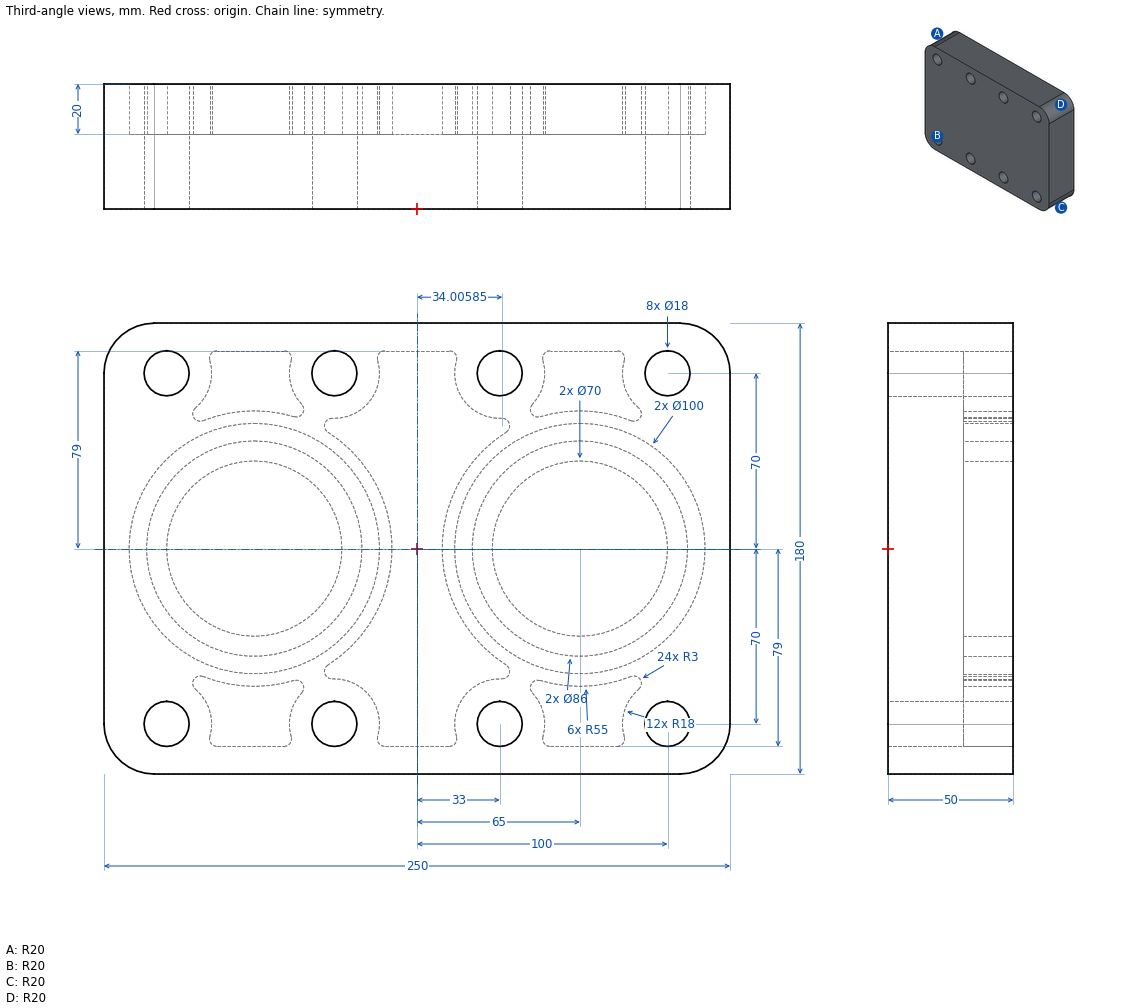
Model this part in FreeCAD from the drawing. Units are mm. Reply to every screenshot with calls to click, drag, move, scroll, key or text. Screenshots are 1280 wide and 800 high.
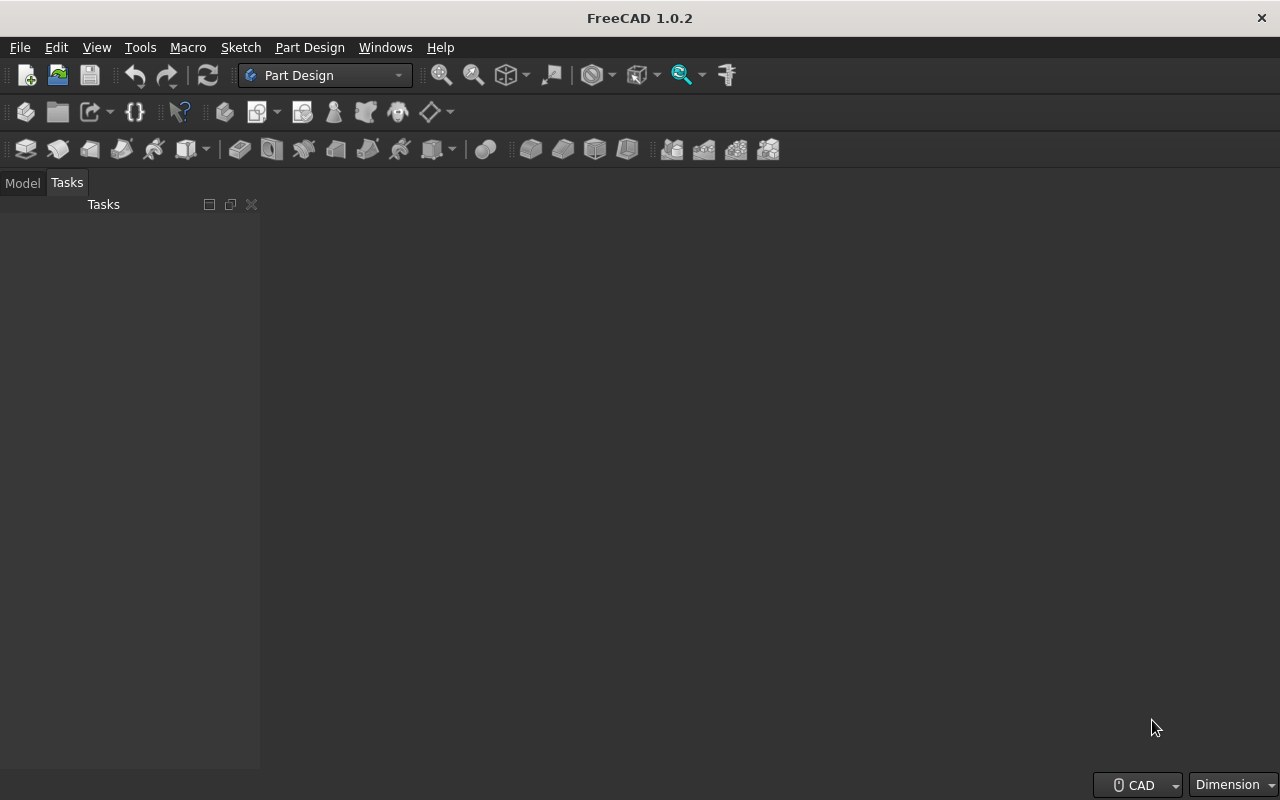
click(26, 76)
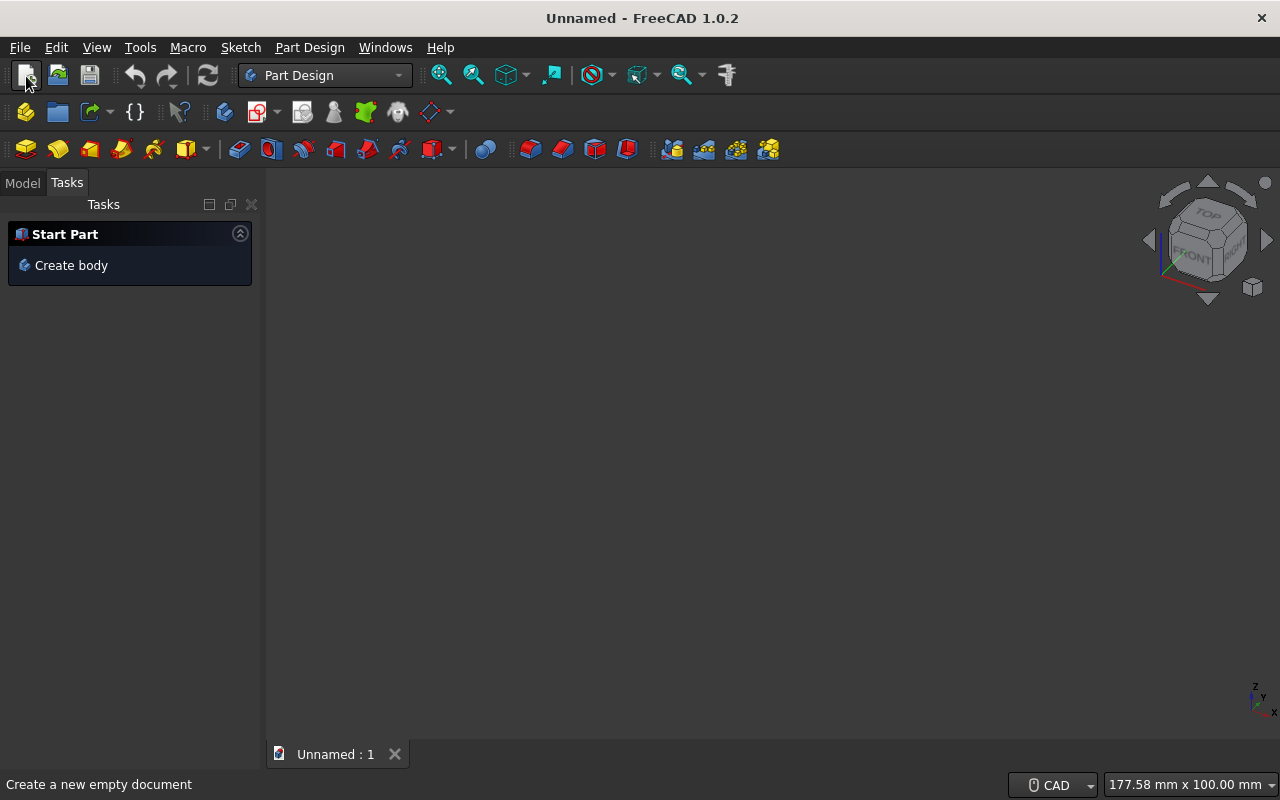
click(258, 112)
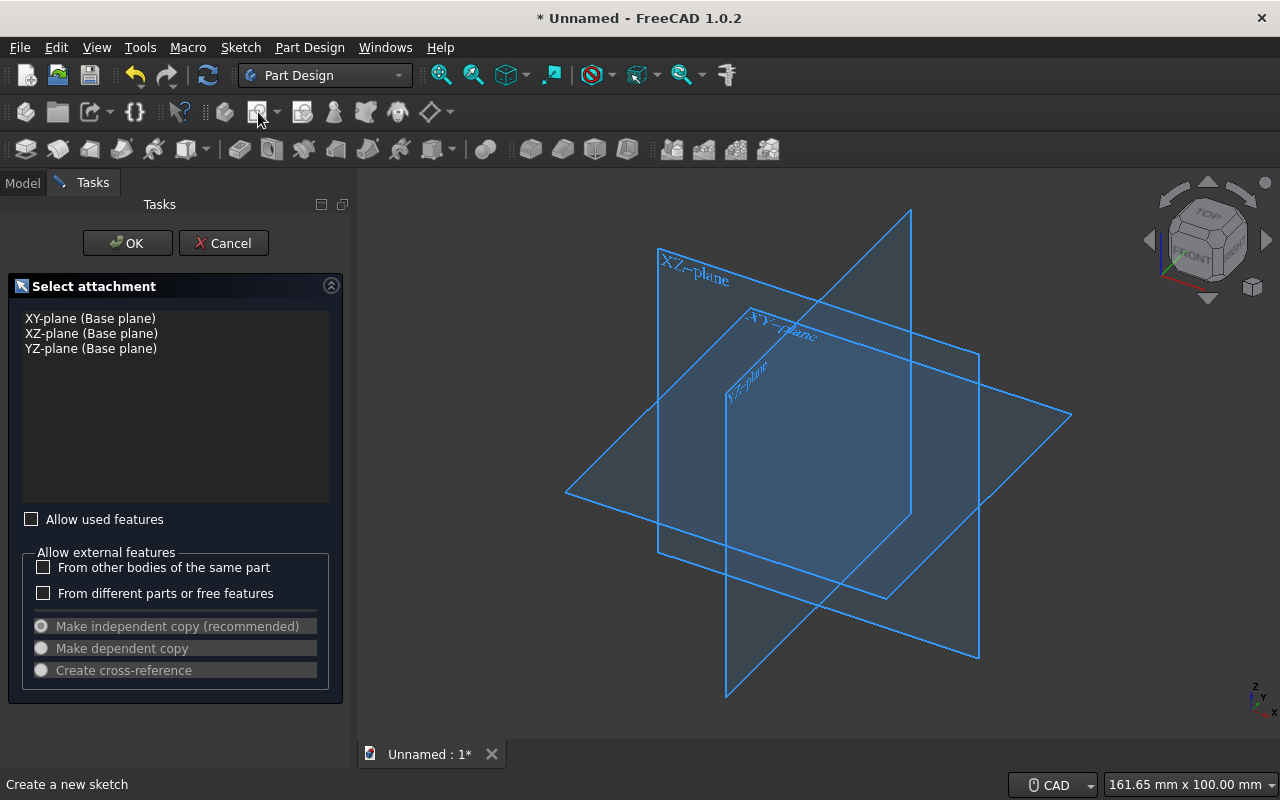
click(82, 334)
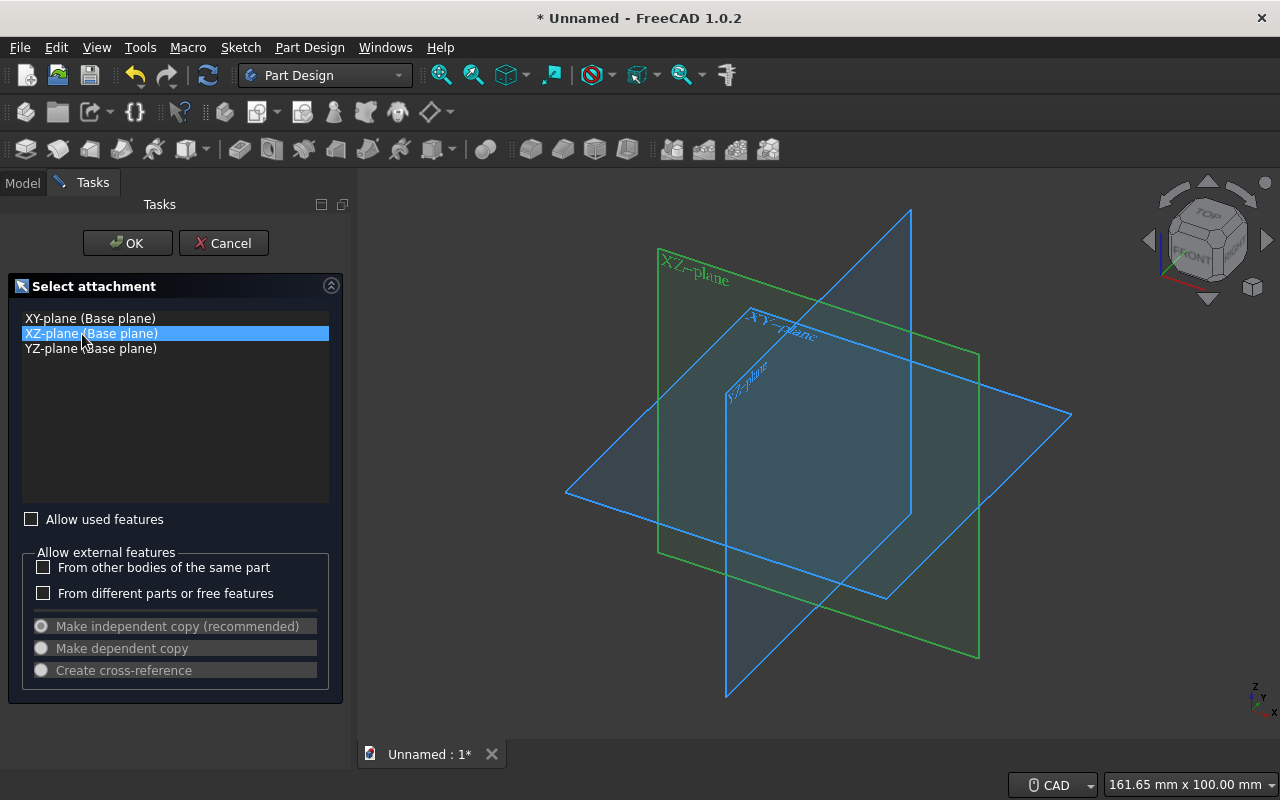
click(128, 243)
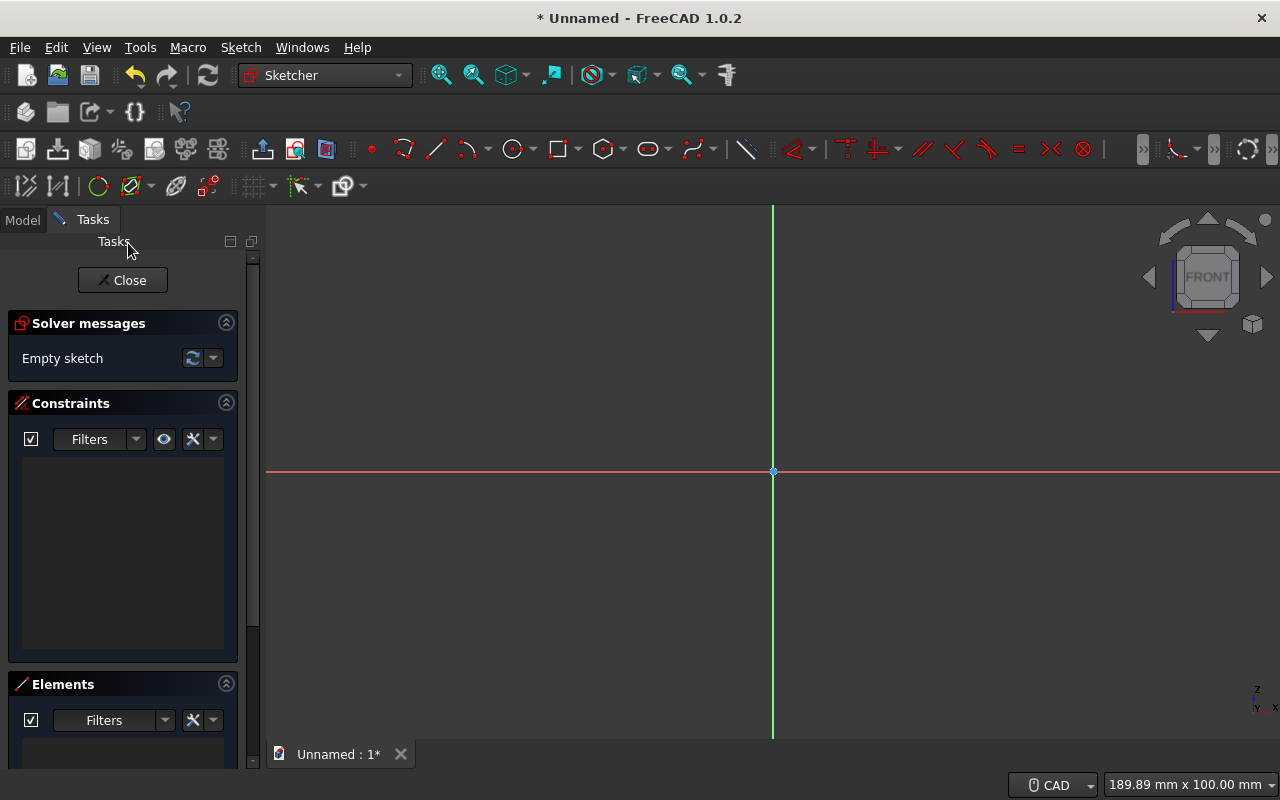
scroll(665, 472, down, 5)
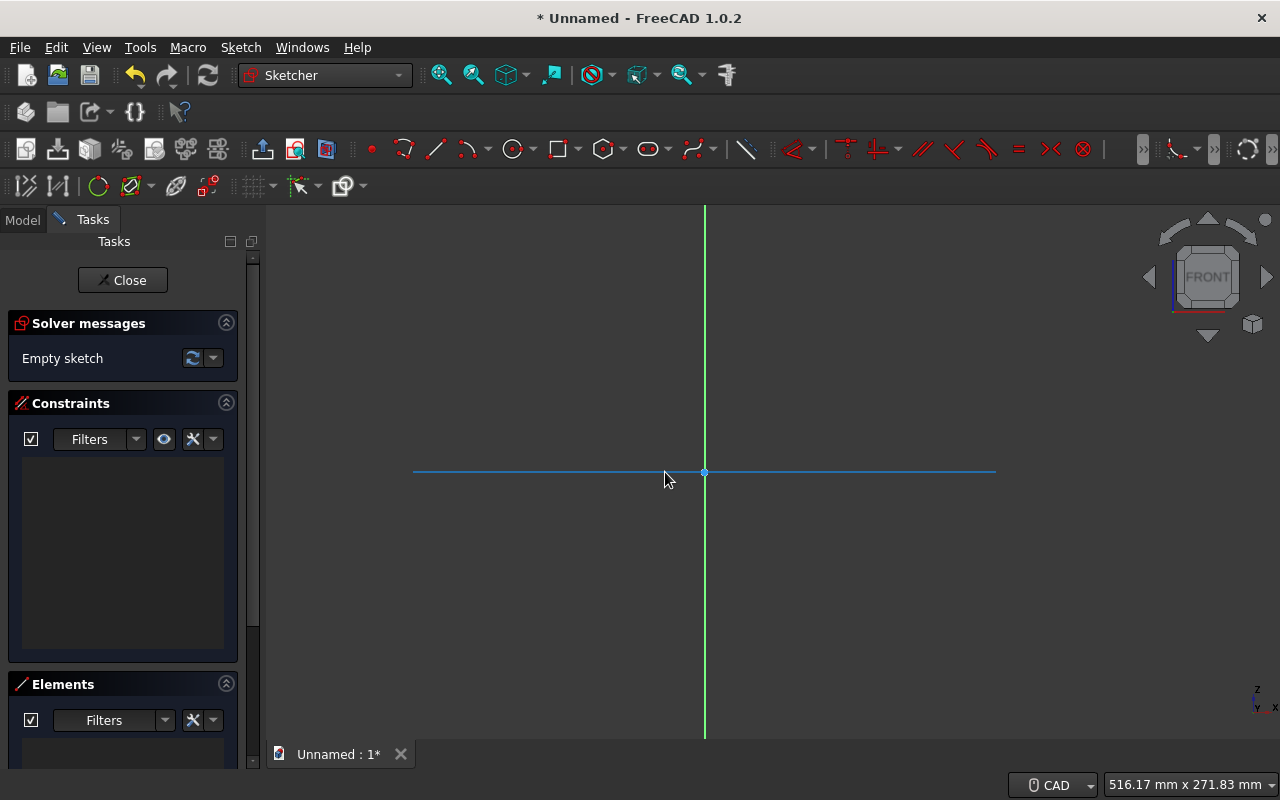
key(g)
key(v)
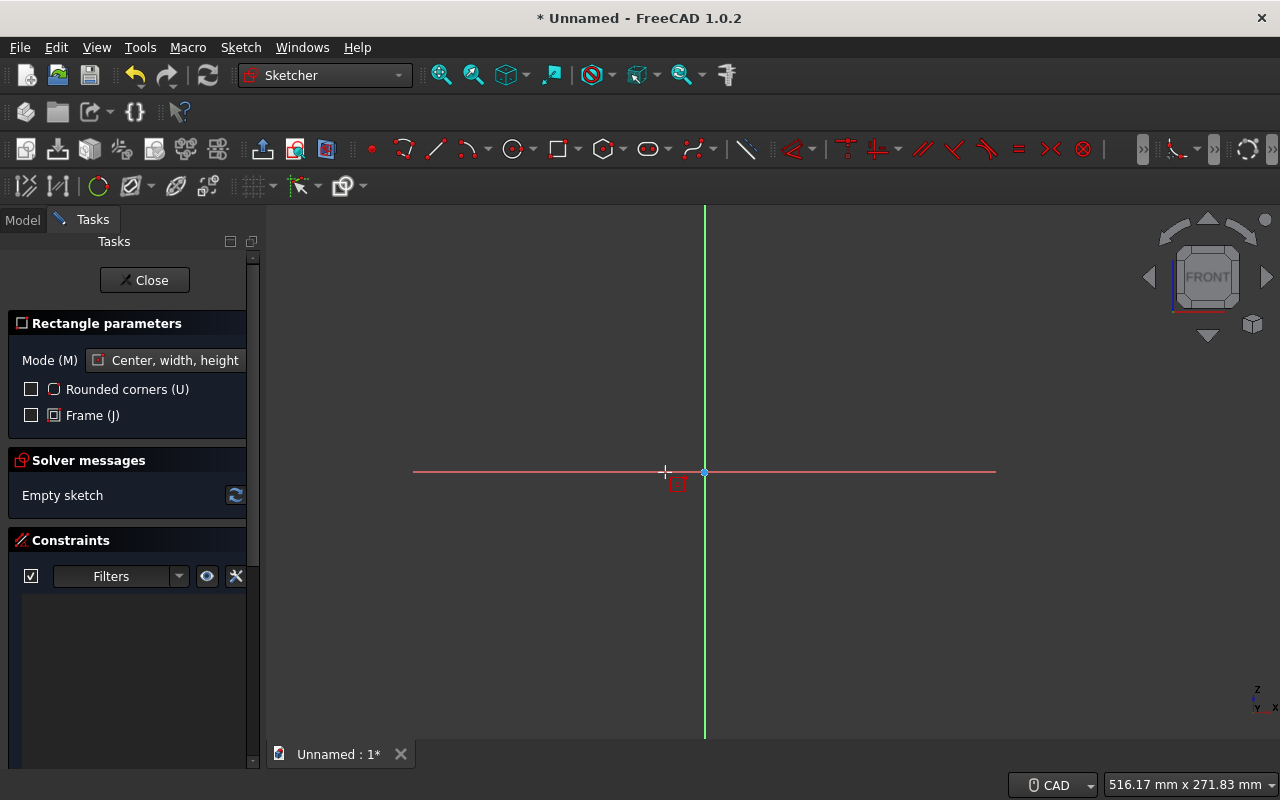
click(705, 472)
move(951, 296)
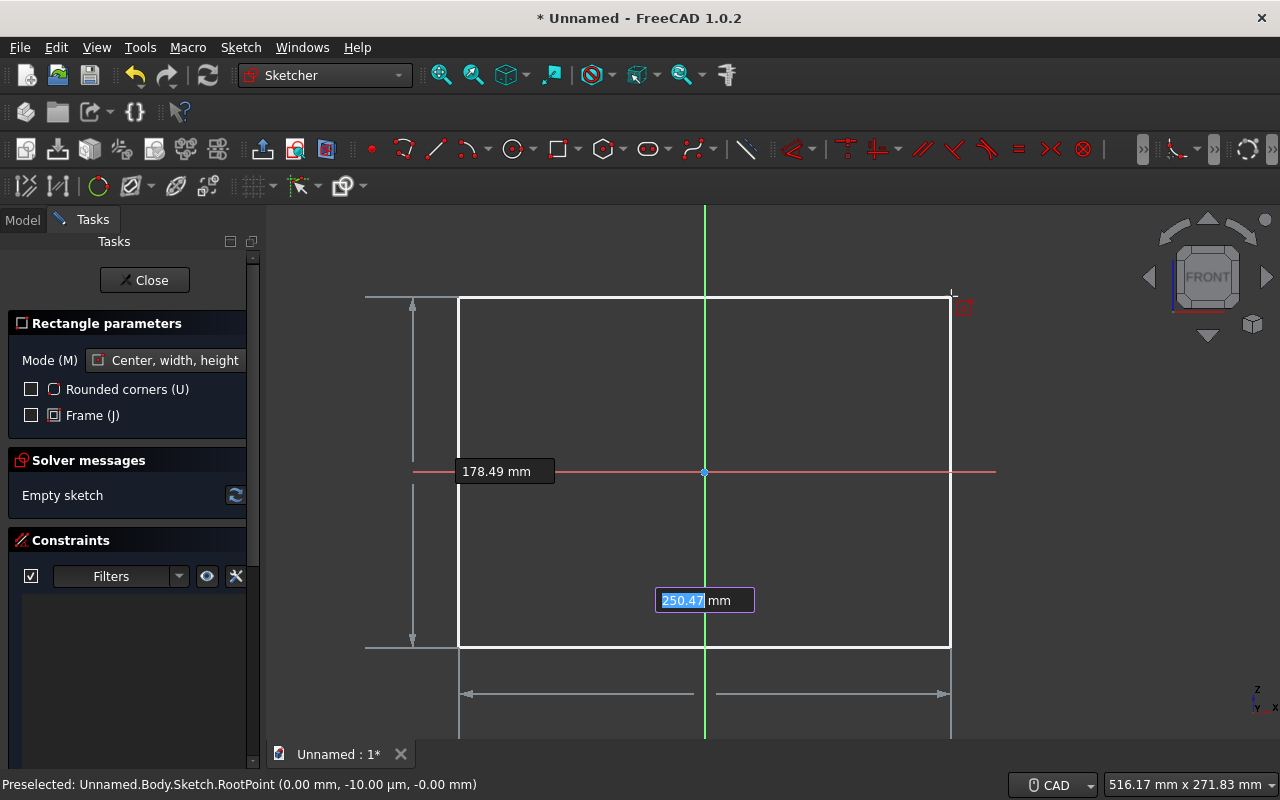
text(250)
key(Tab)
text(180)
key(Return)
key(Escape)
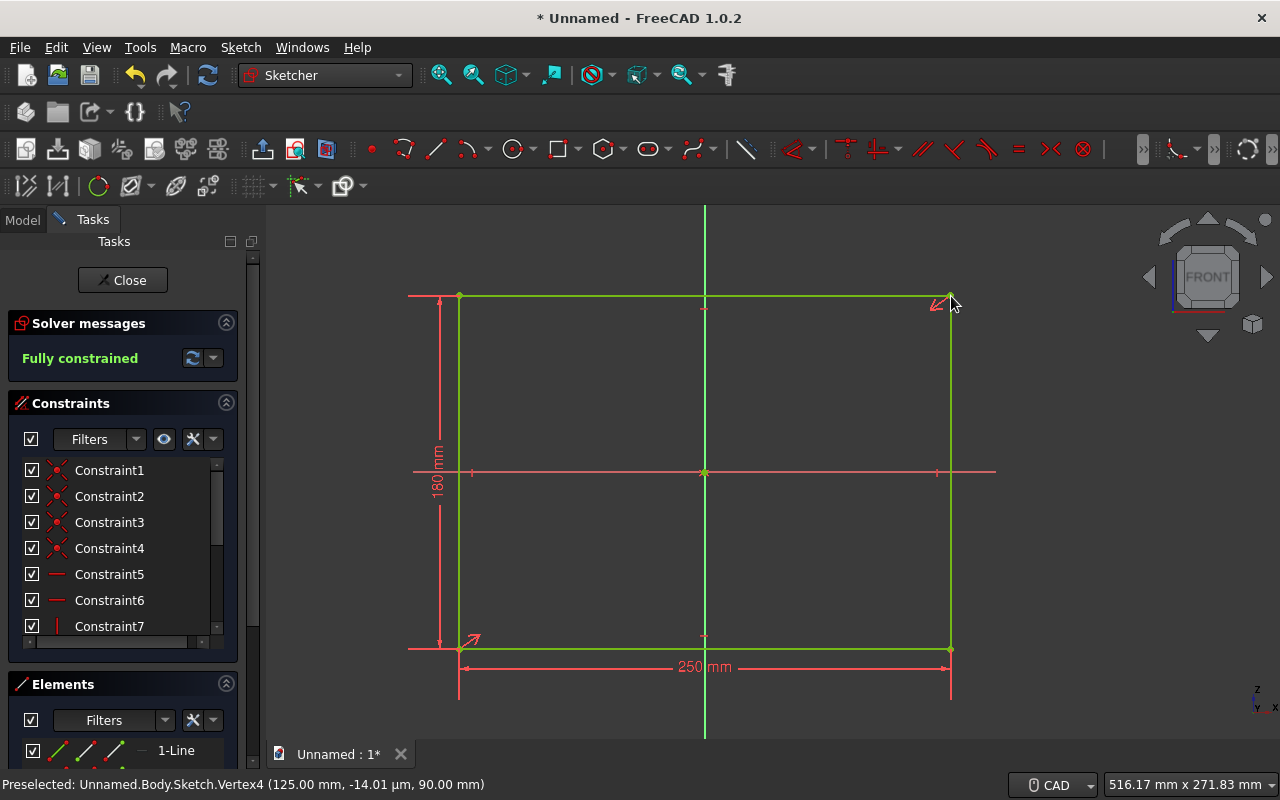
click(123, 280)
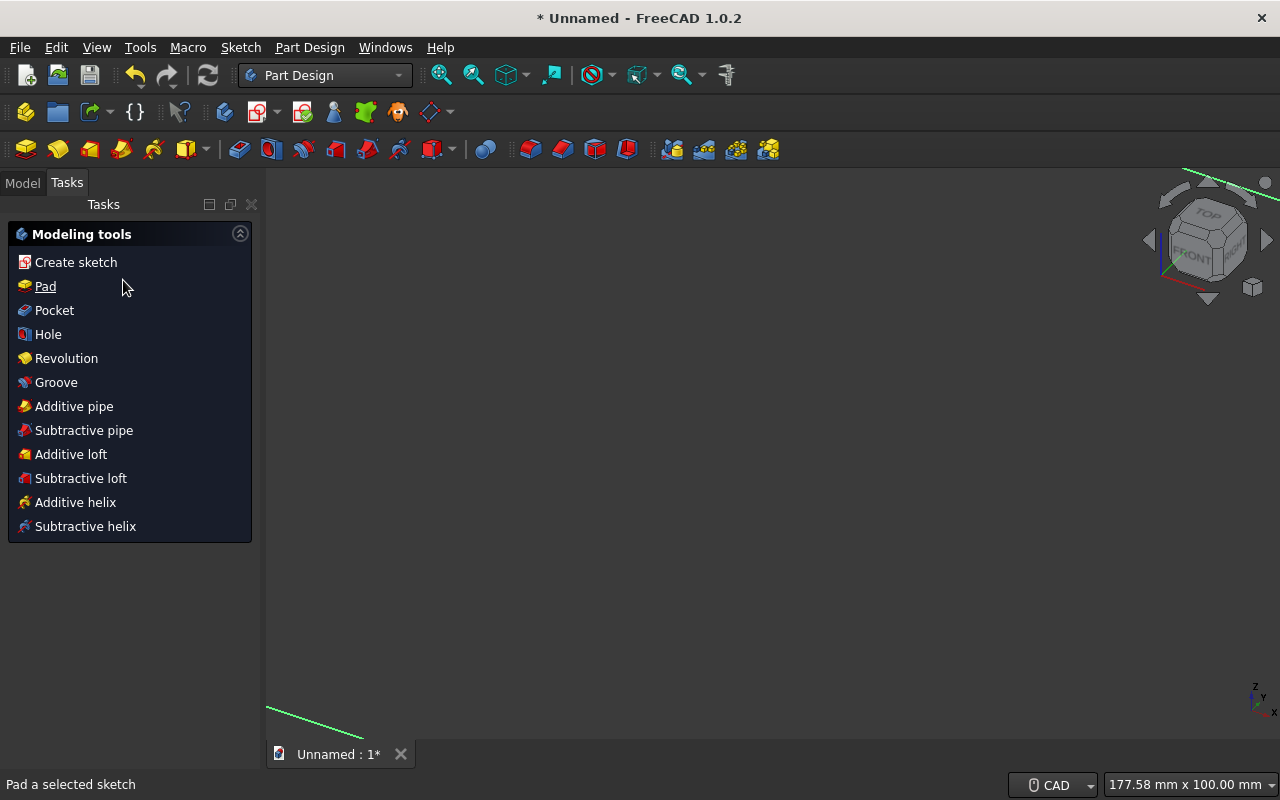
click(26, 150)